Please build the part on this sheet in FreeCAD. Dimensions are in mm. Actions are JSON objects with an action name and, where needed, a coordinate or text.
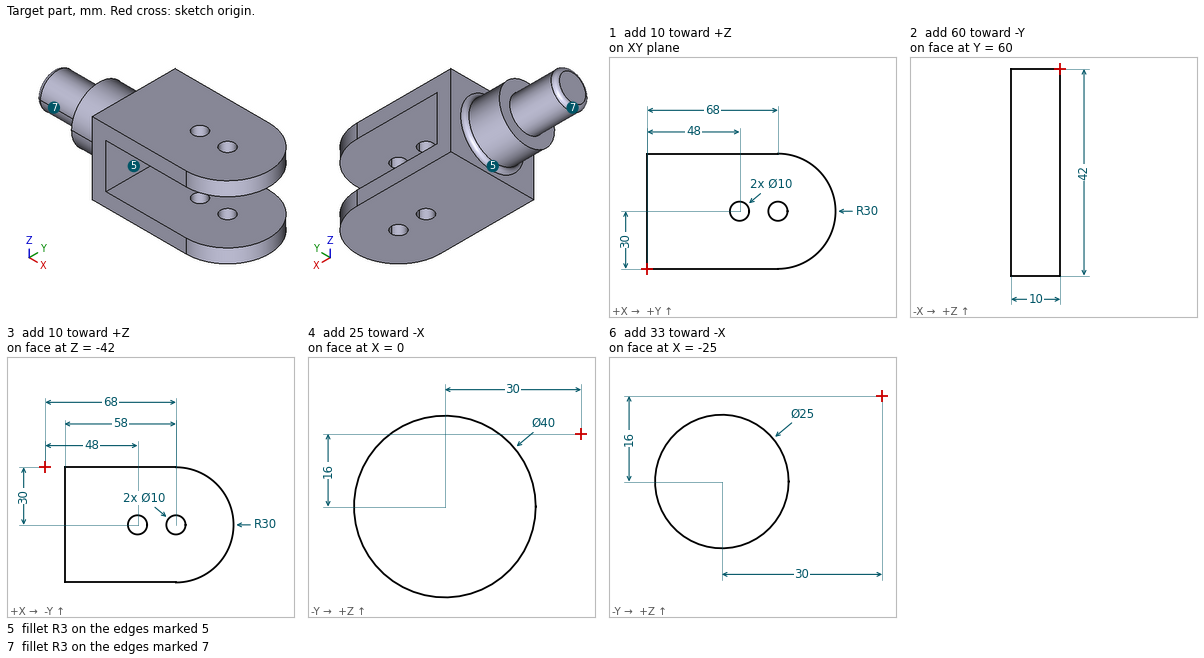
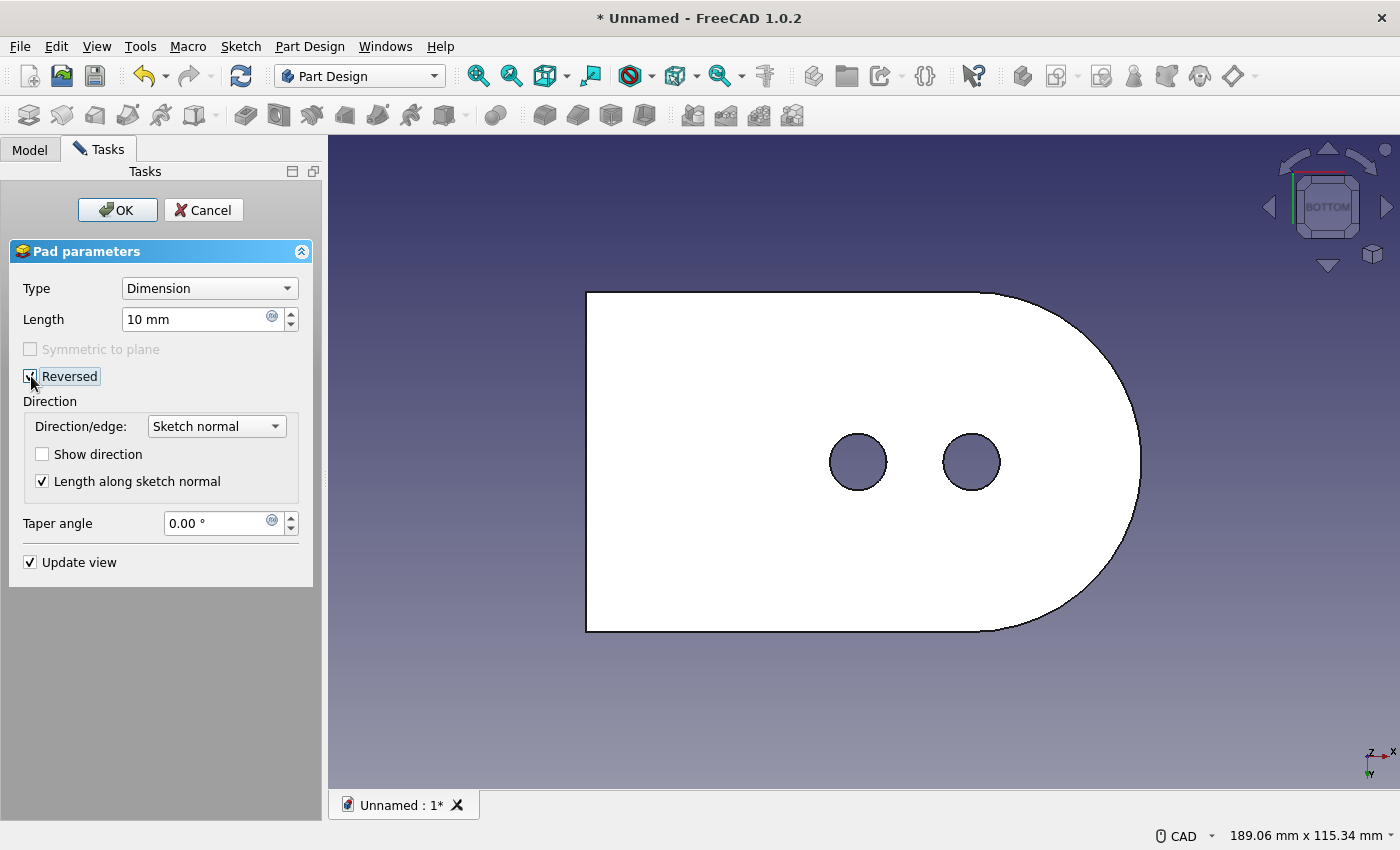
{"action": "left_click", "coordinate": [118, 210]}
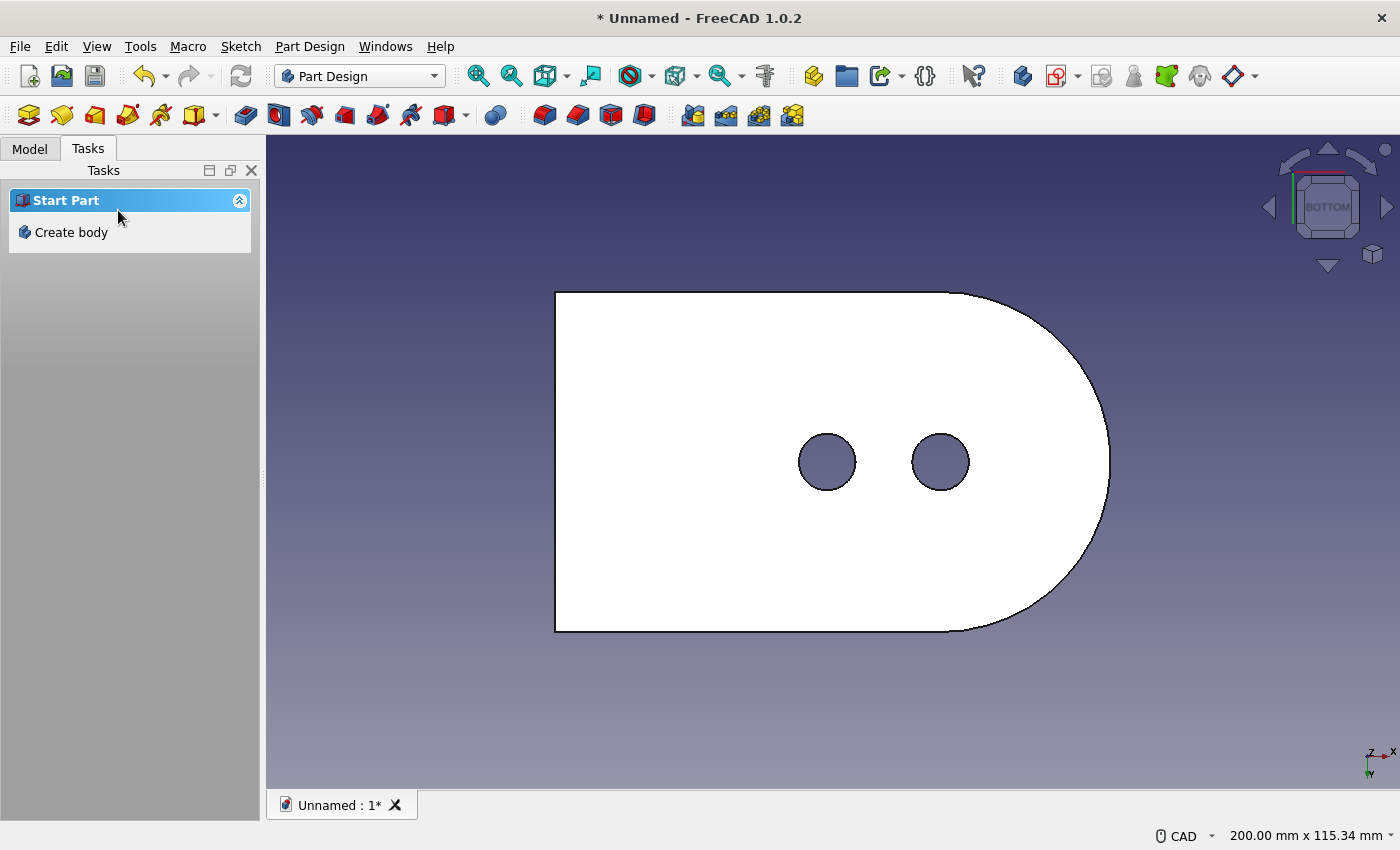
{"action": "key", "text": "6"}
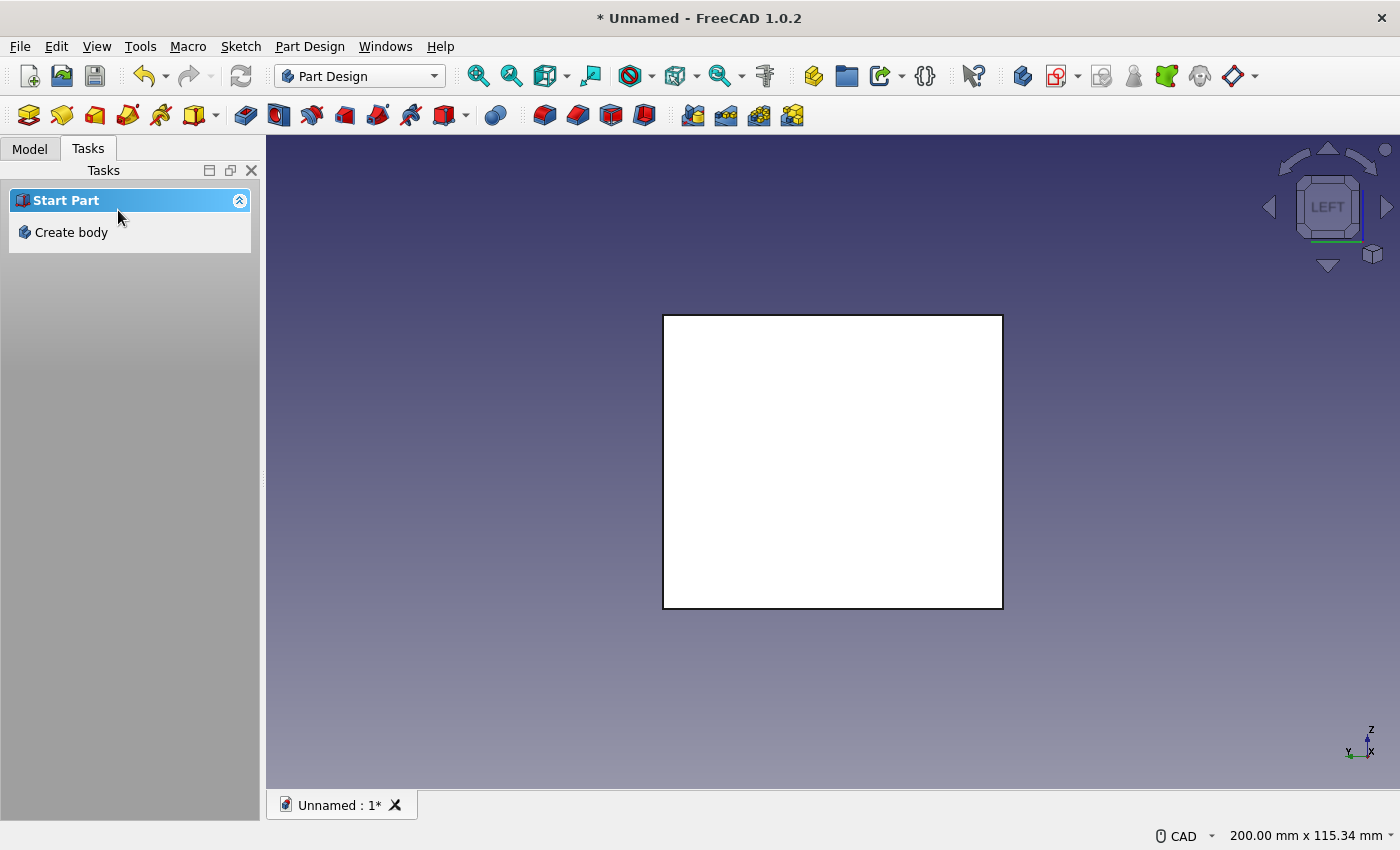
{"action": "key", "text": "v f"}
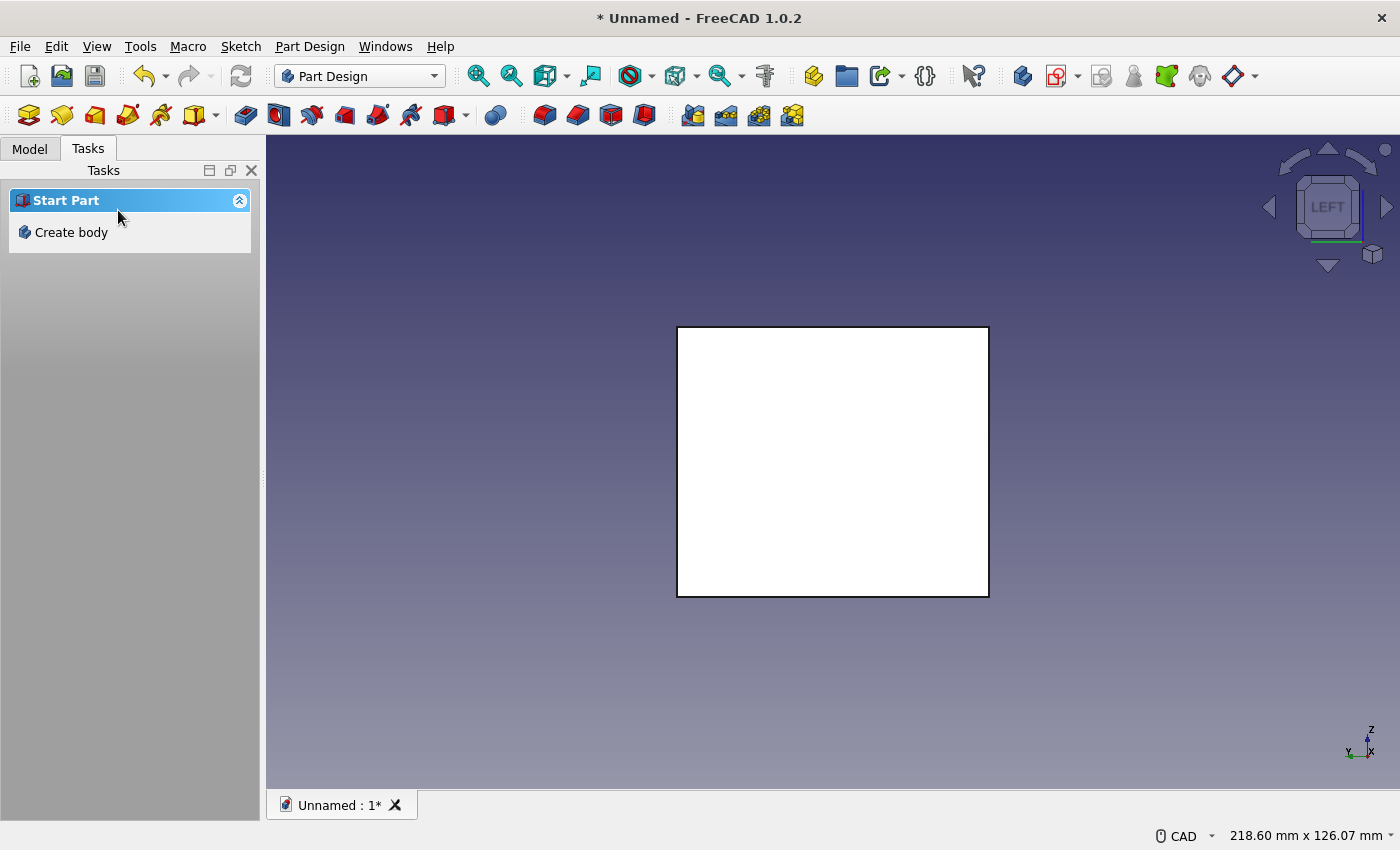
{"action": "left_click", "coordinate": [833, 461]}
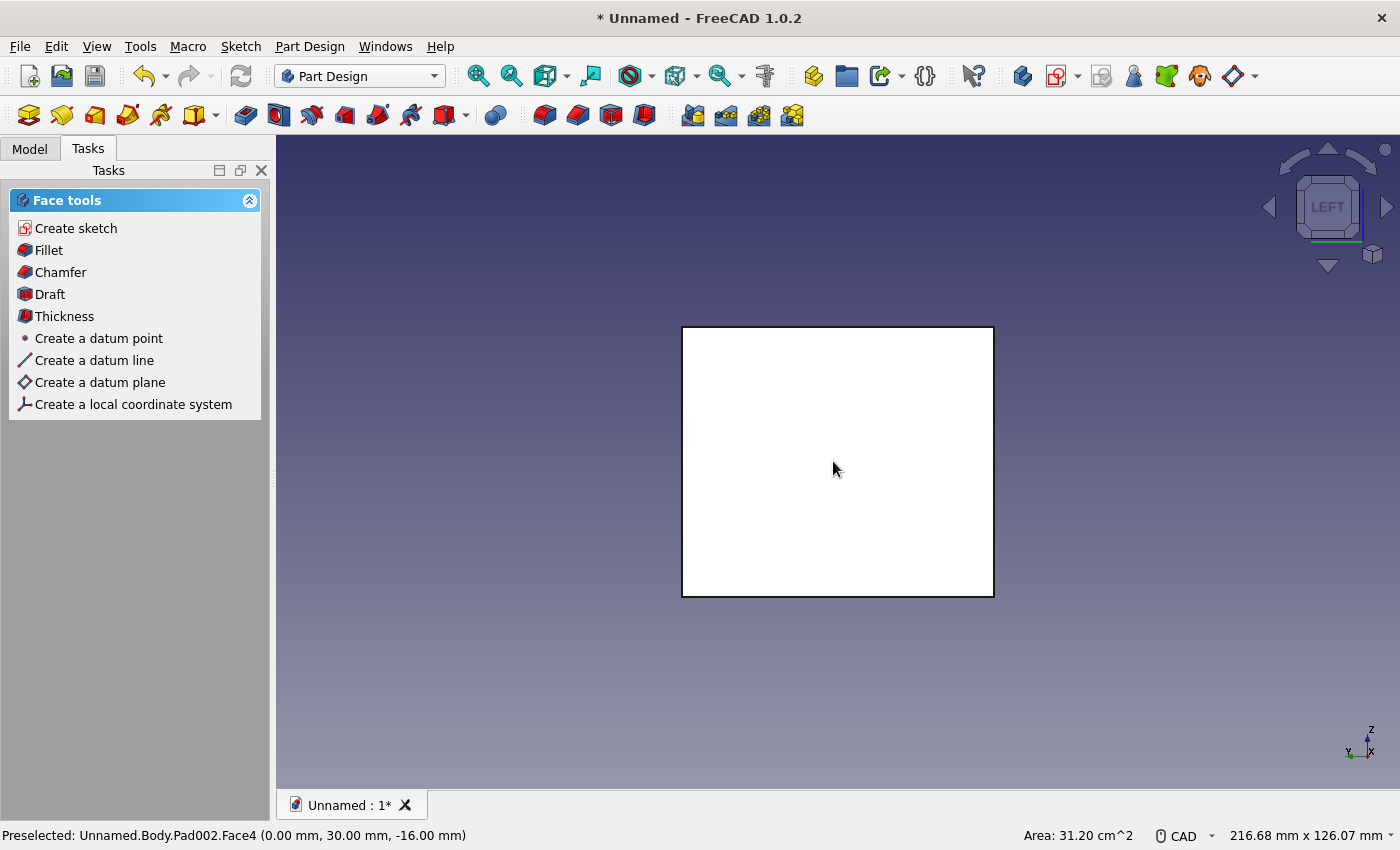
{"action": "left_click", "coordinate": [1056, 76]}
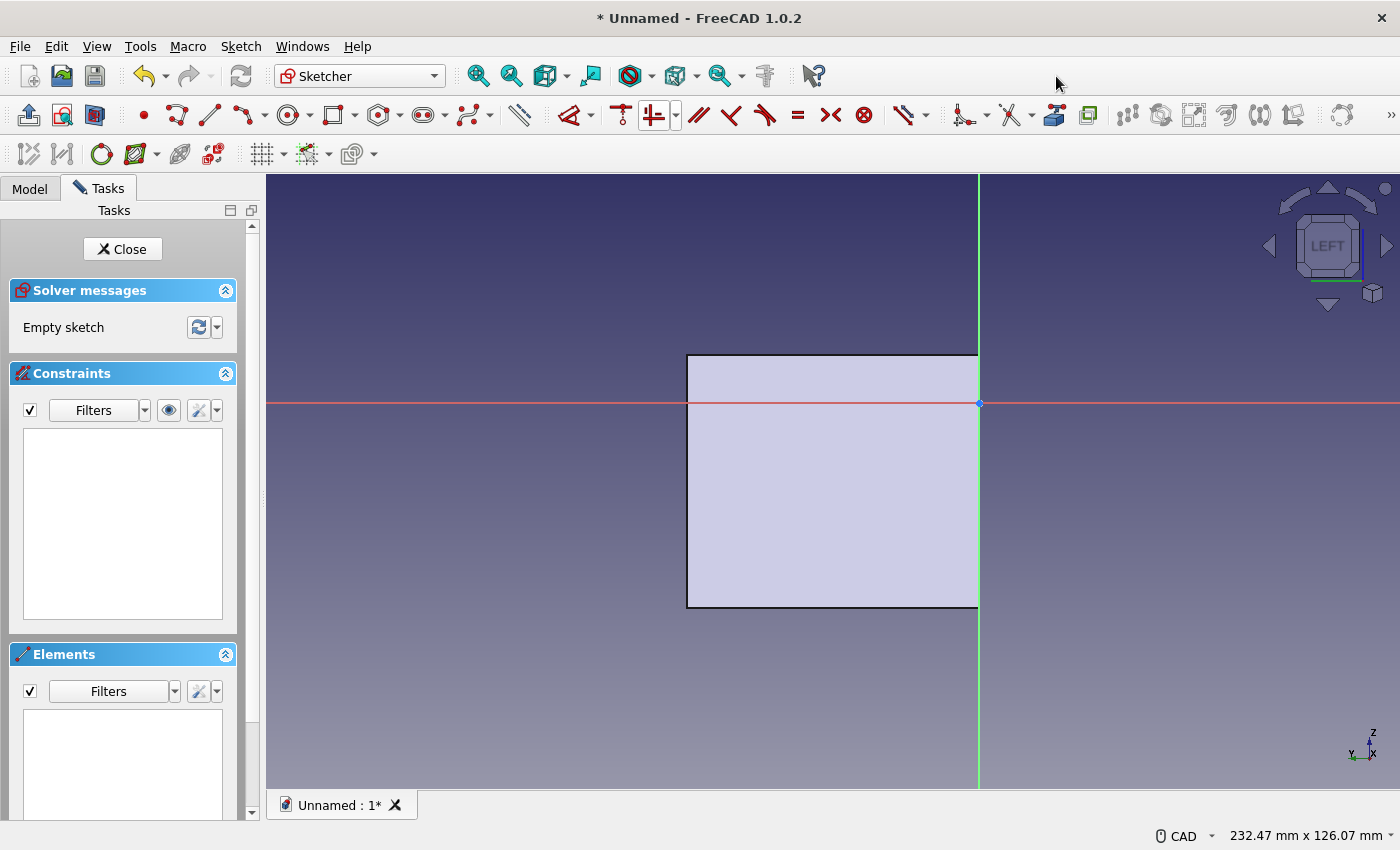
{"action": "scroll", "coordinate": [933, 482], "scroll_direction": "up", "scroll_amount": 4}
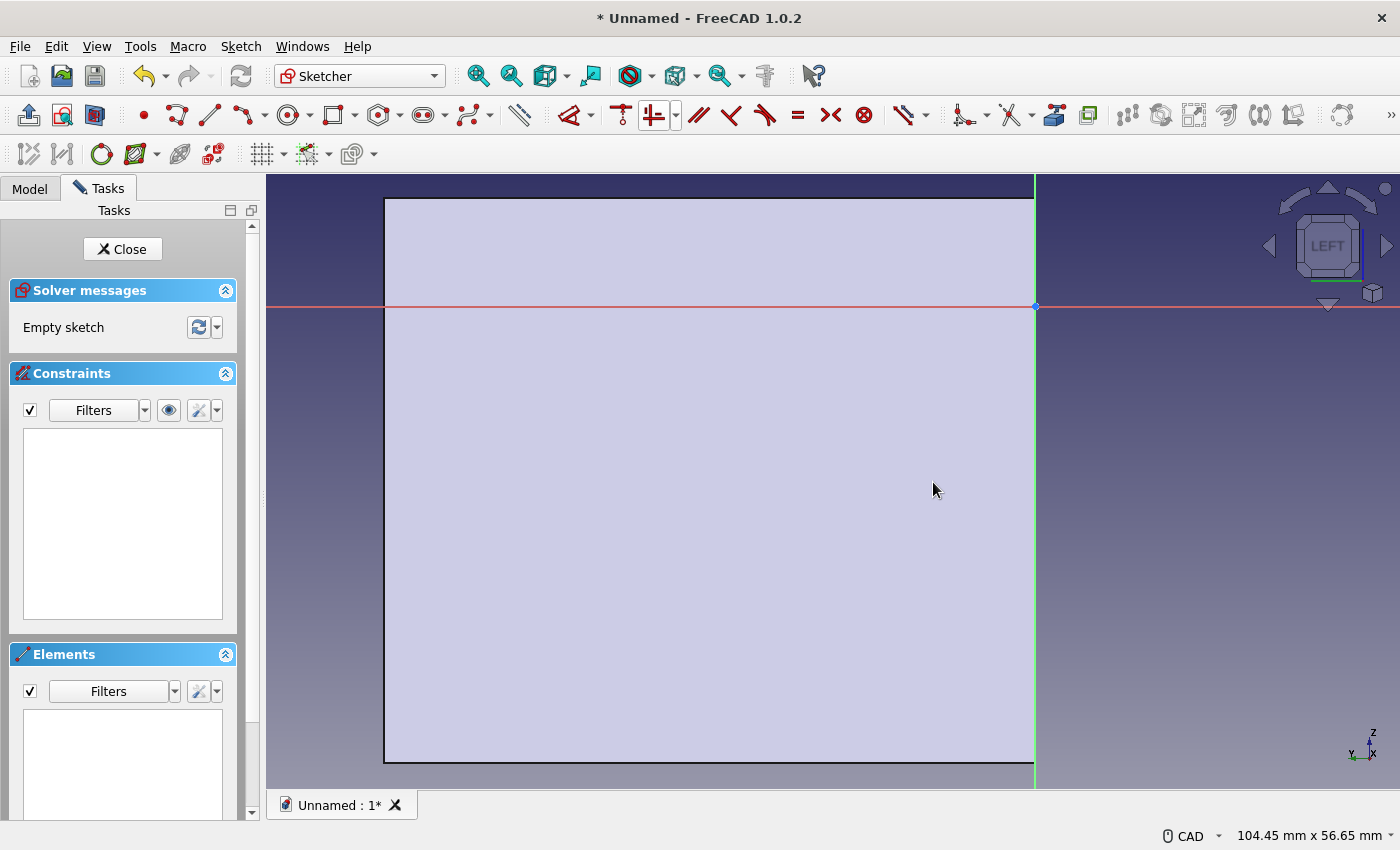
{"action": "key", "text": "g c"}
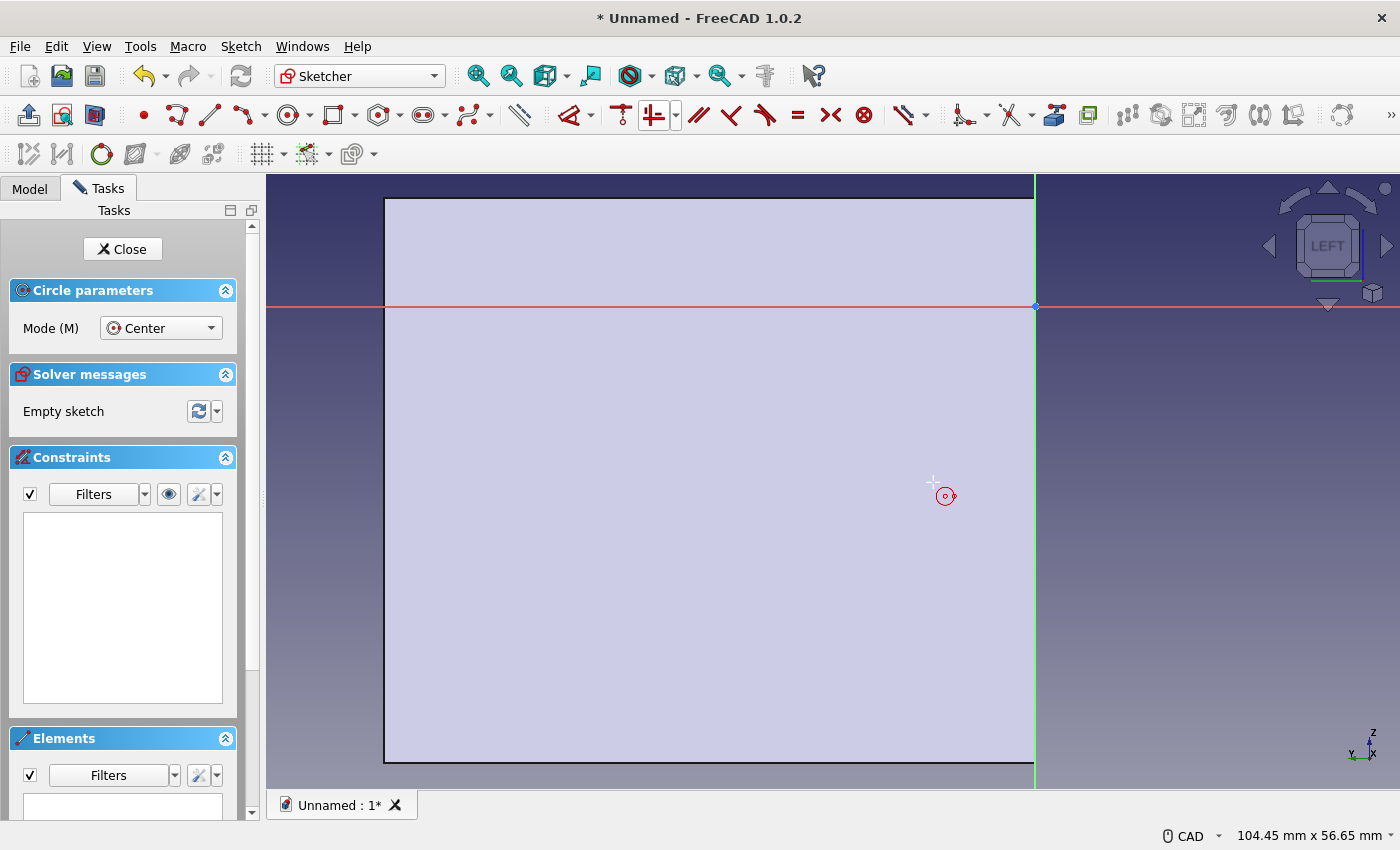
{"action": "left_click", "coordinate": [710, 480]}
{"action": "mouse_move", "coordinate": [863, 327]}